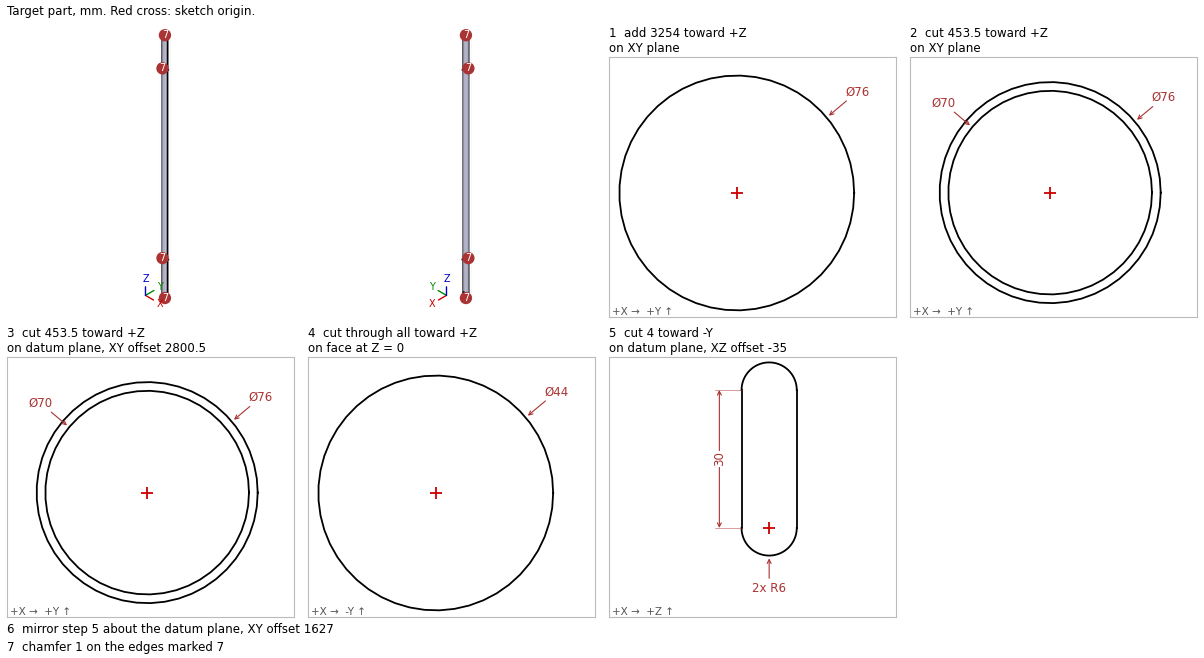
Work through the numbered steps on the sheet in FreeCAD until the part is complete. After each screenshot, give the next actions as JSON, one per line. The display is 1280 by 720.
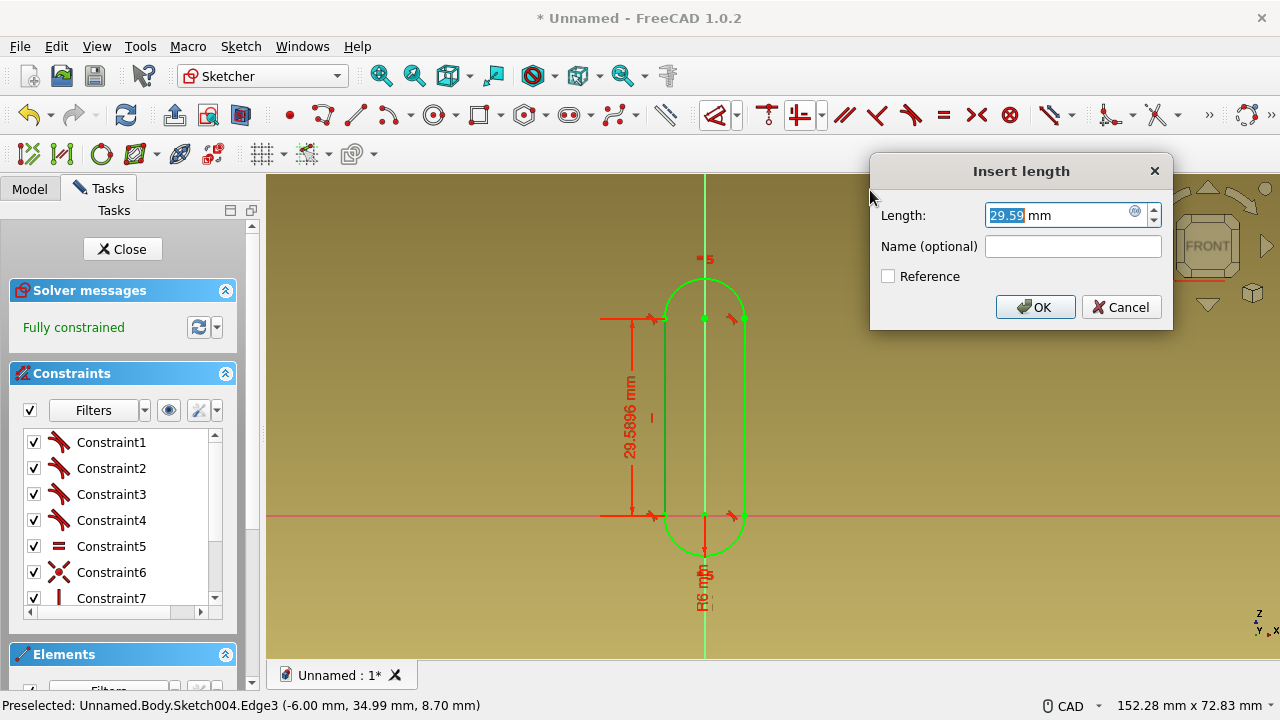
{"action": "type", "text": "30"}
{"action": "key", "text": "Return"}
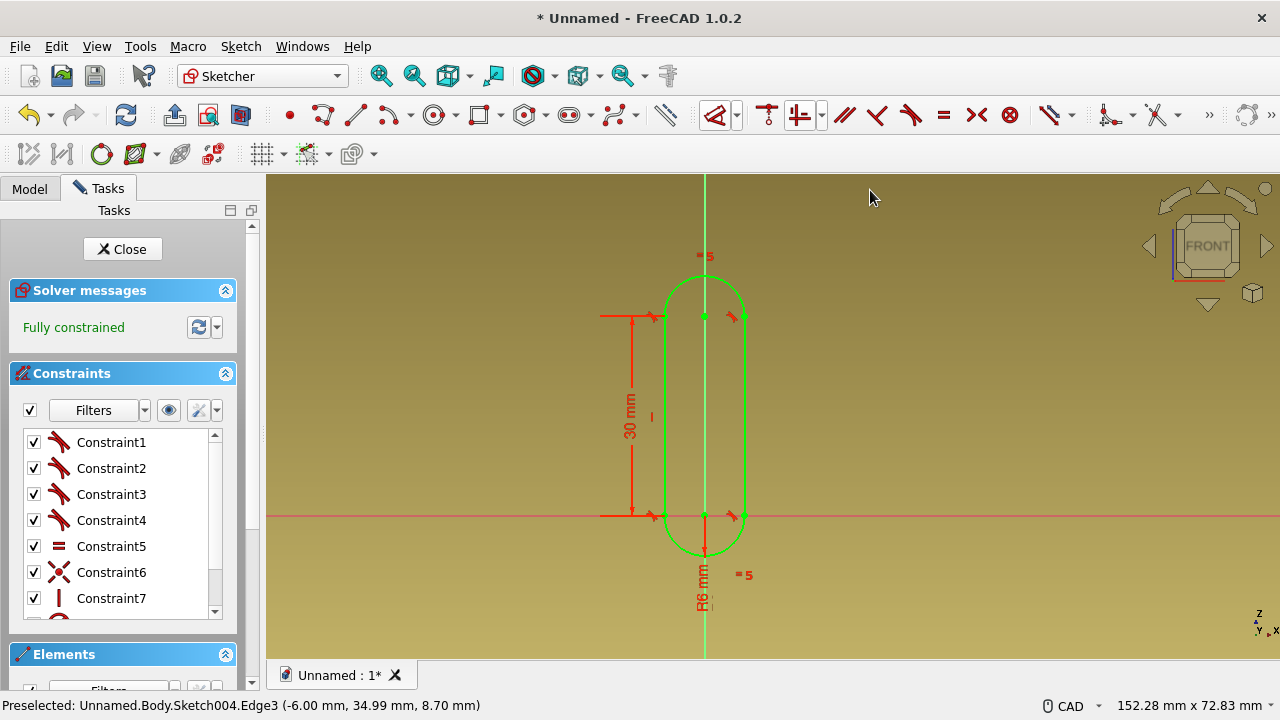
{"action": "left_click", "coordinate": [123, 249]}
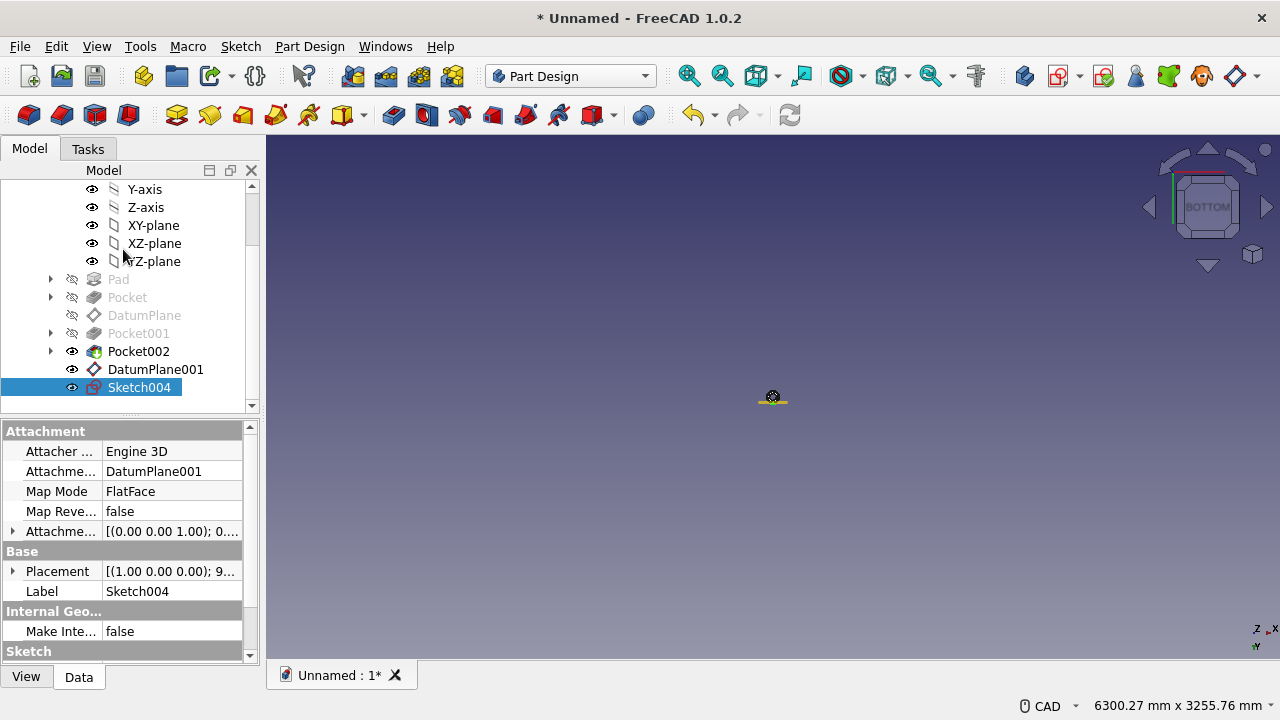
{"action": "left_click", "coordinate": [394, 116]}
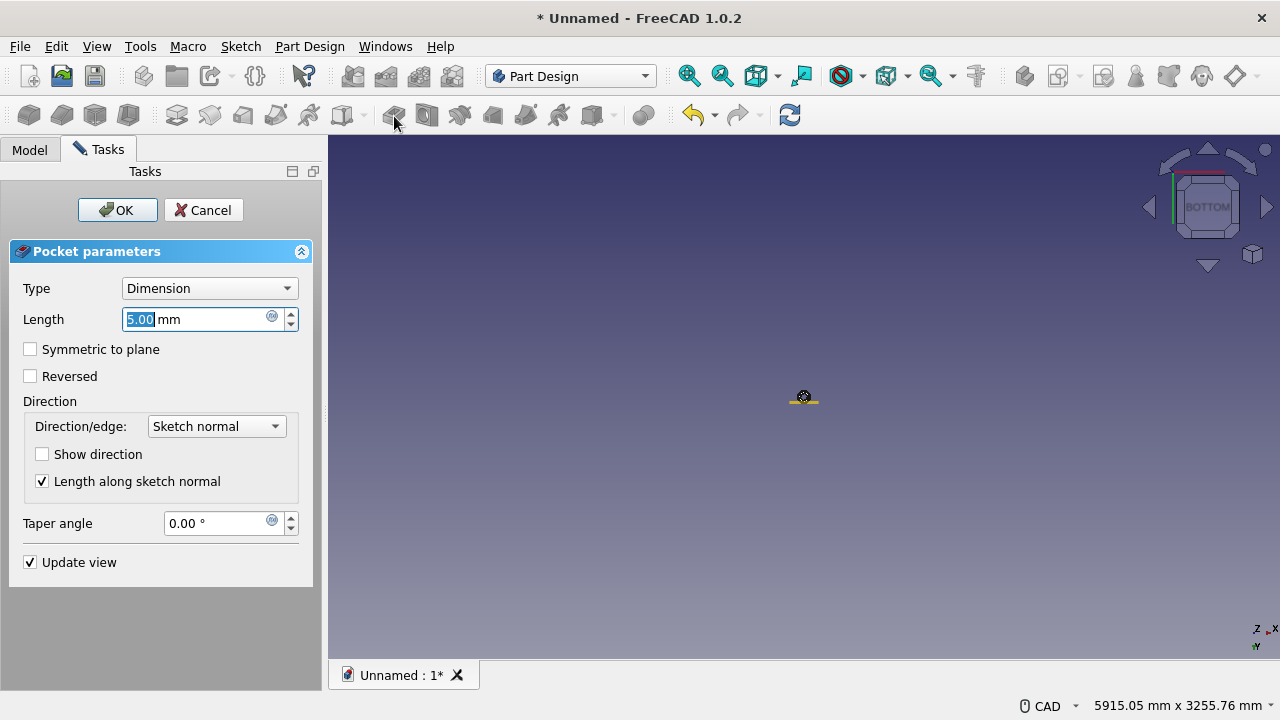
{"action": "type", "text": "4"}
{"action": "key", "text": "Tab"}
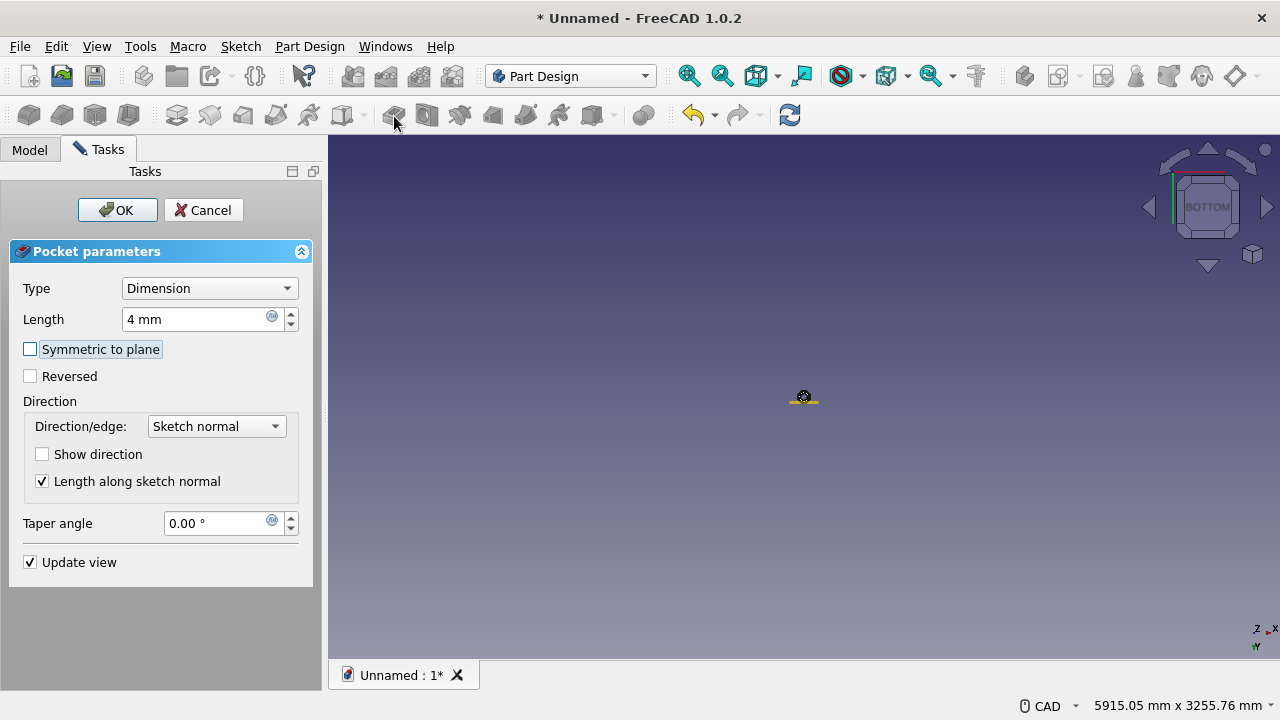
{"action": "left_click", "coordinate": [31, 376]}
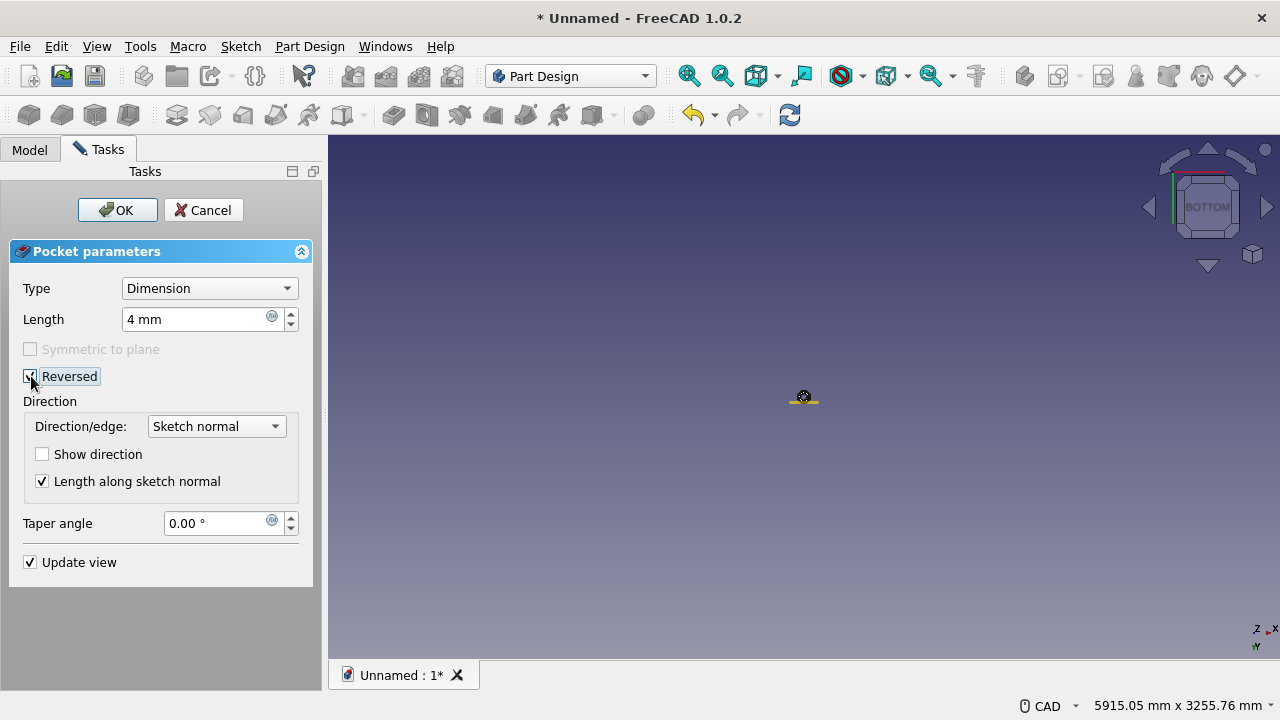
{"action": "left_click", "coordinate": [118, 210]}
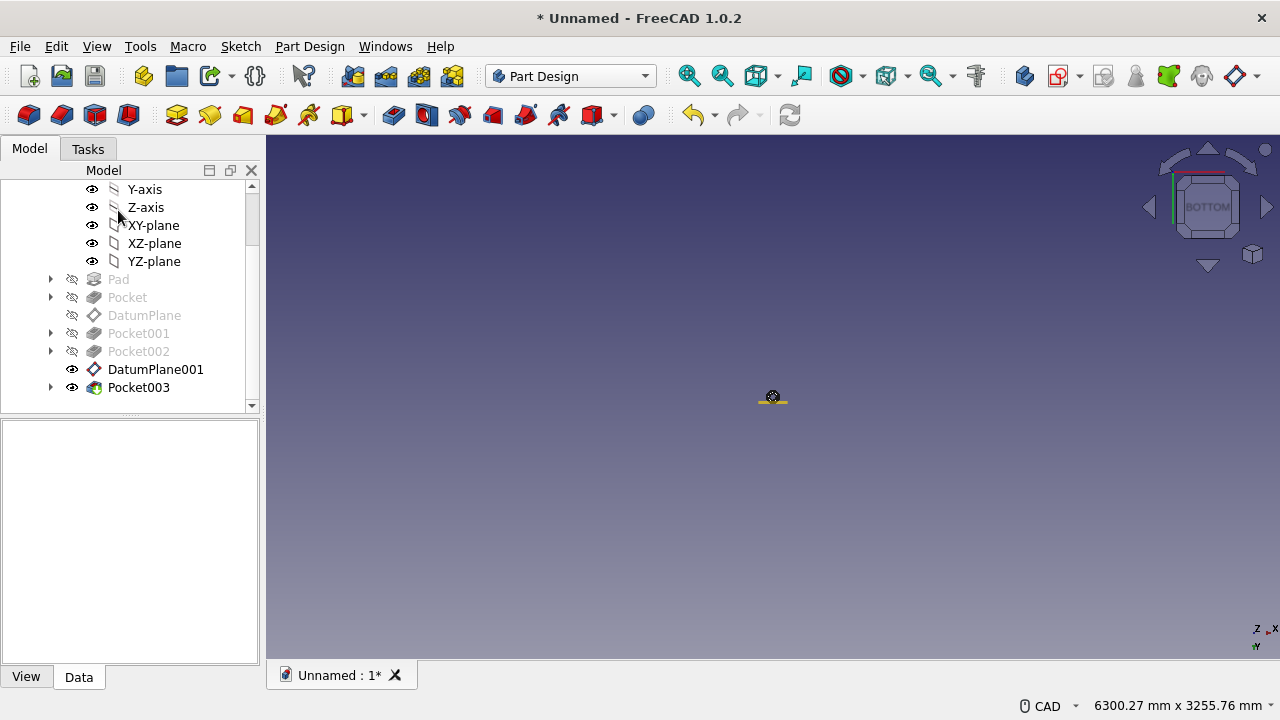
{"action": "left_click", "coordinate": [117, 369]}
{"action": "key", "text": "space"}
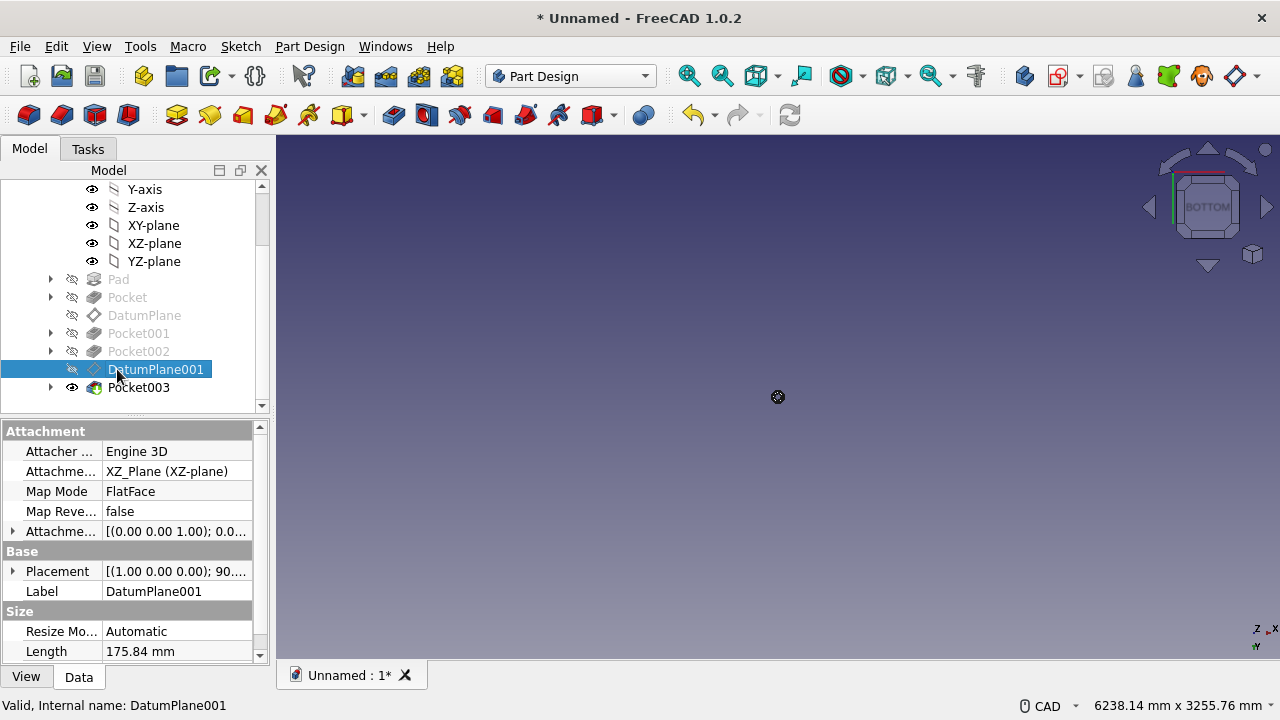
{"action": "left_click", "coordinate": [690, 76]}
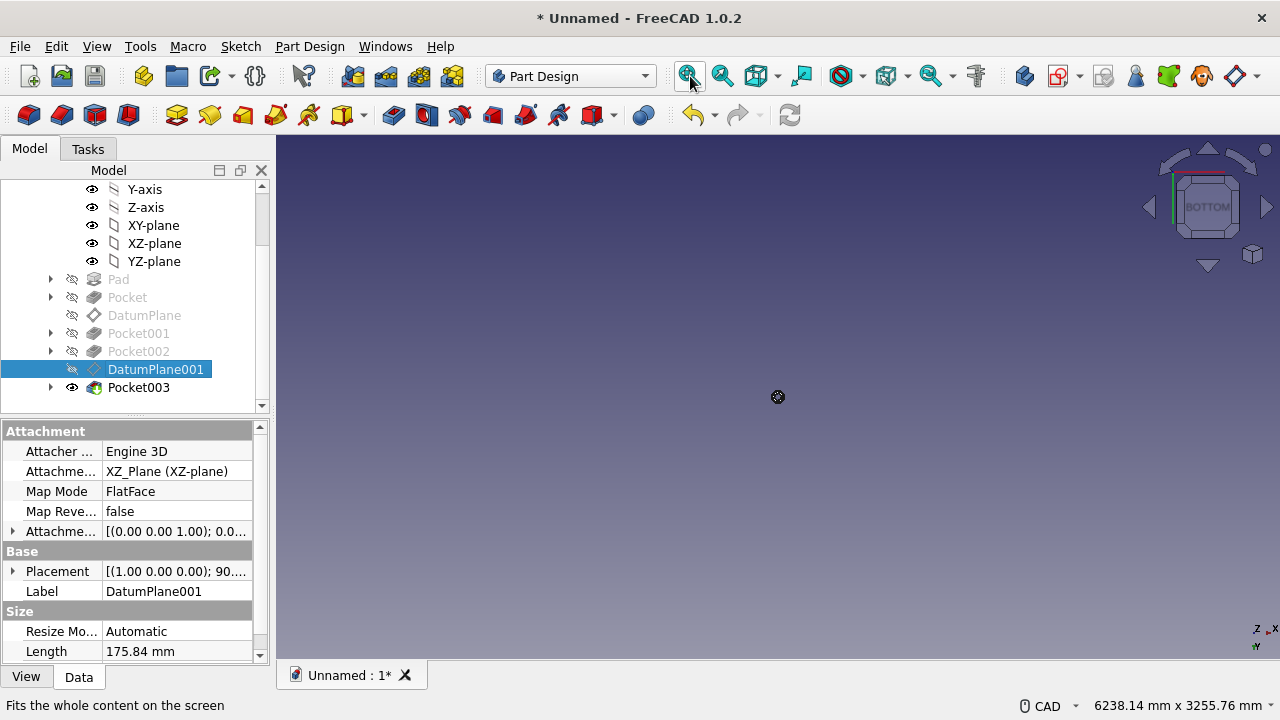
{"action": "scroll", "coordinate": [161, 293], "scroll_direction": "down", "scroll_amount": 3}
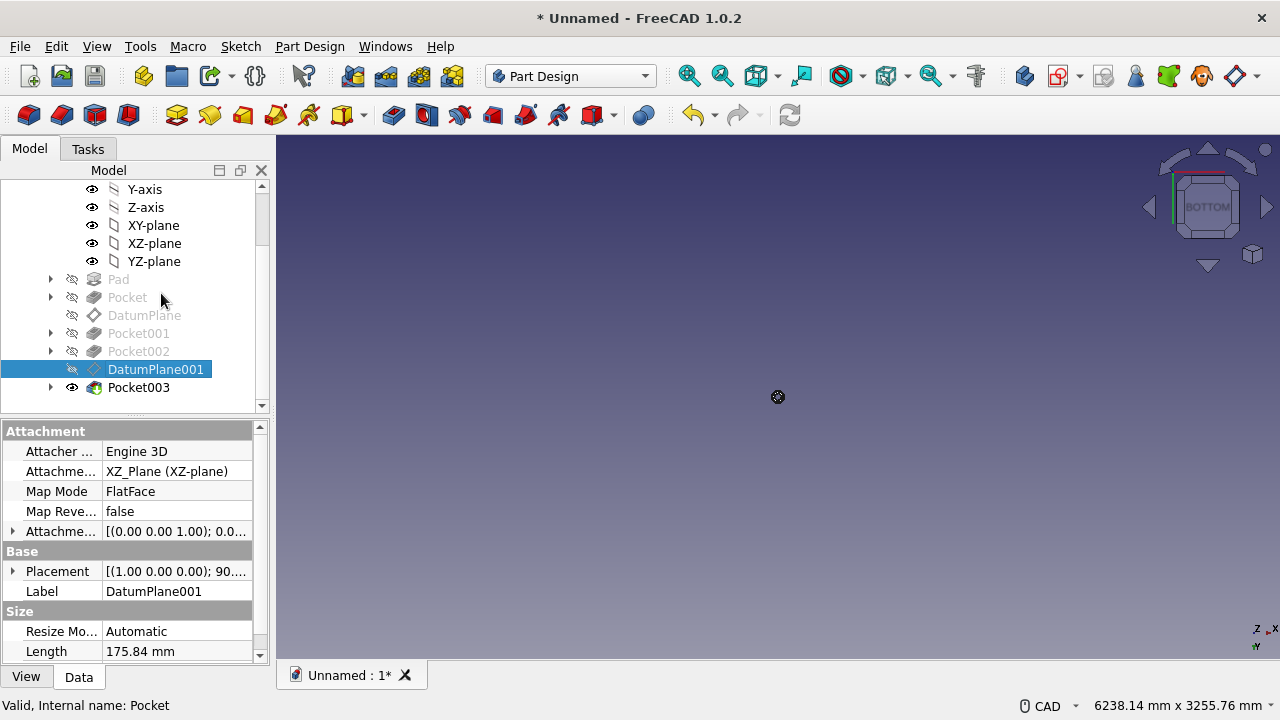
{"action": "scroll", "coordinate": [161, 293], "scroll_direction": "up", "scroll_amount": 15}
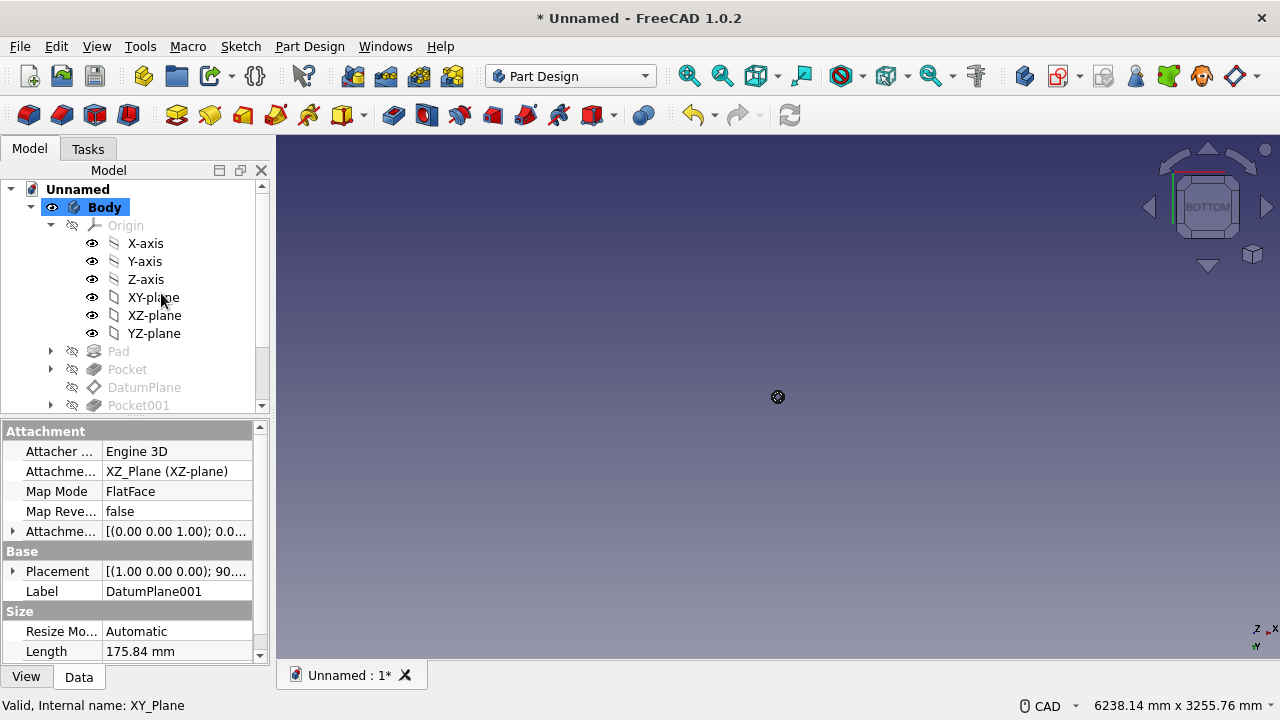
{"action": "left_click", "coordinate": [137, 297]}